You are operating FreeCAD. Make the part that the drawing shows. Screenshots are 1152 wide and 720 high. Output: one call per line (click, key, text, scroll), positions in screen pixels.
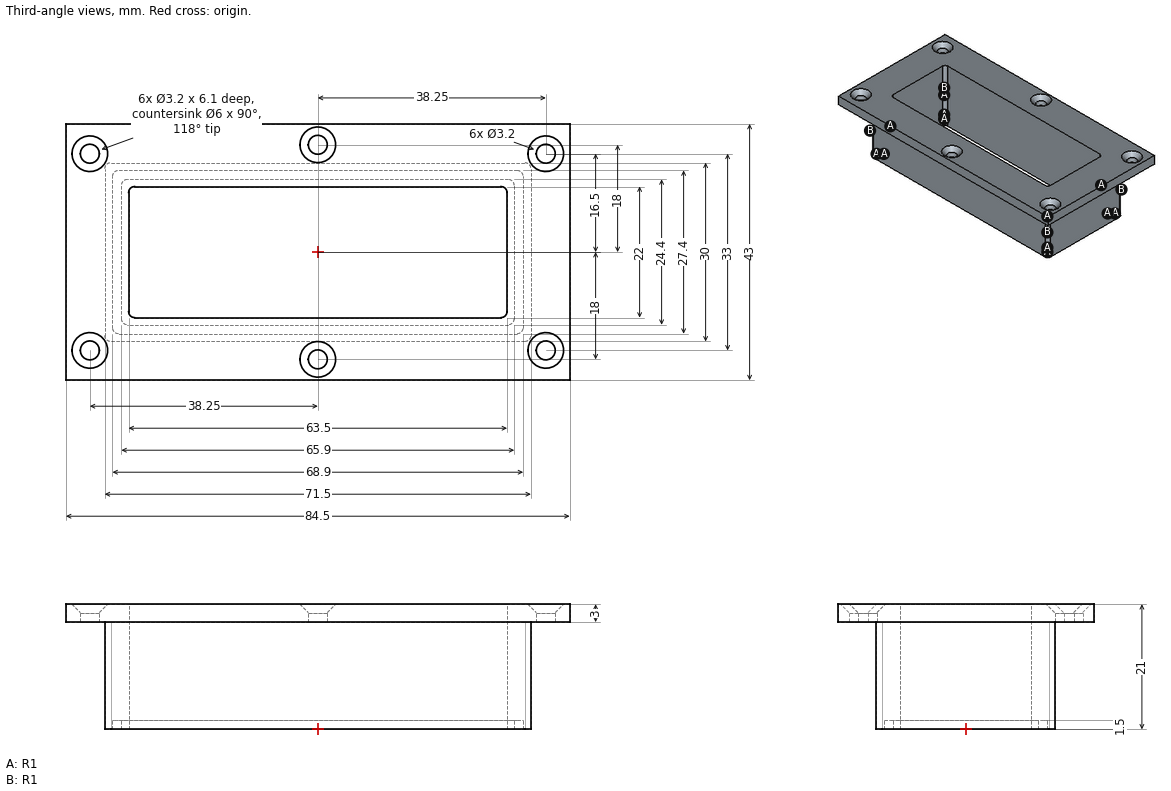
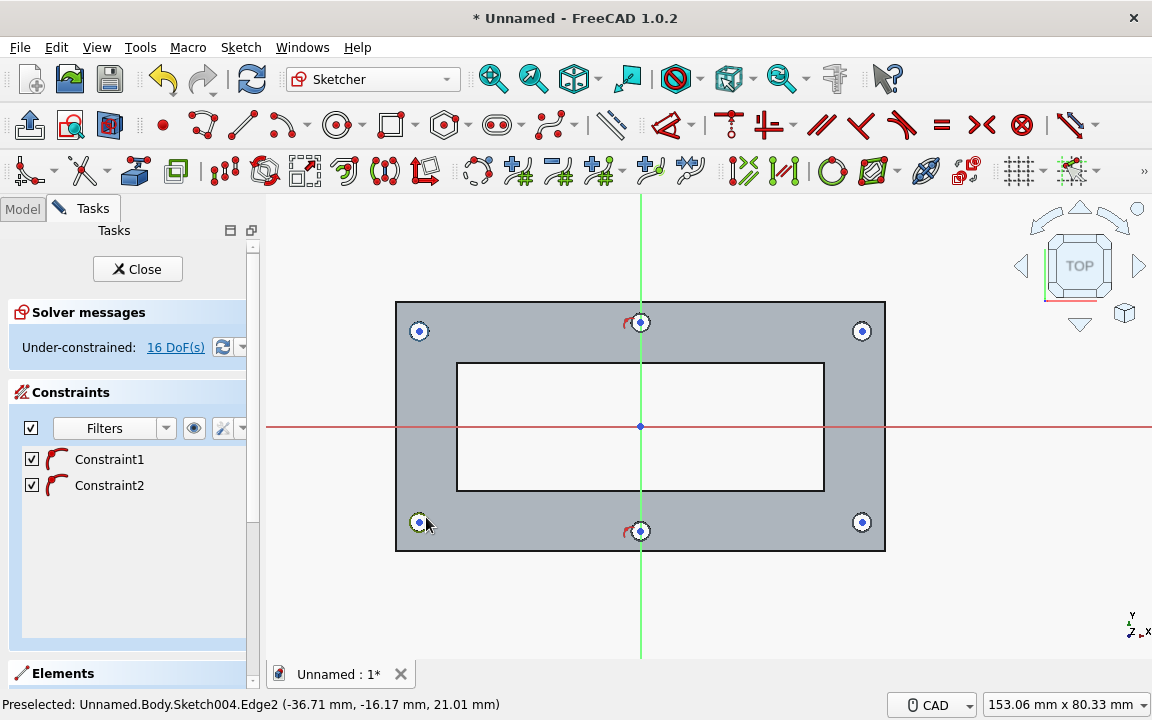
scroll(868, 325, up, 3)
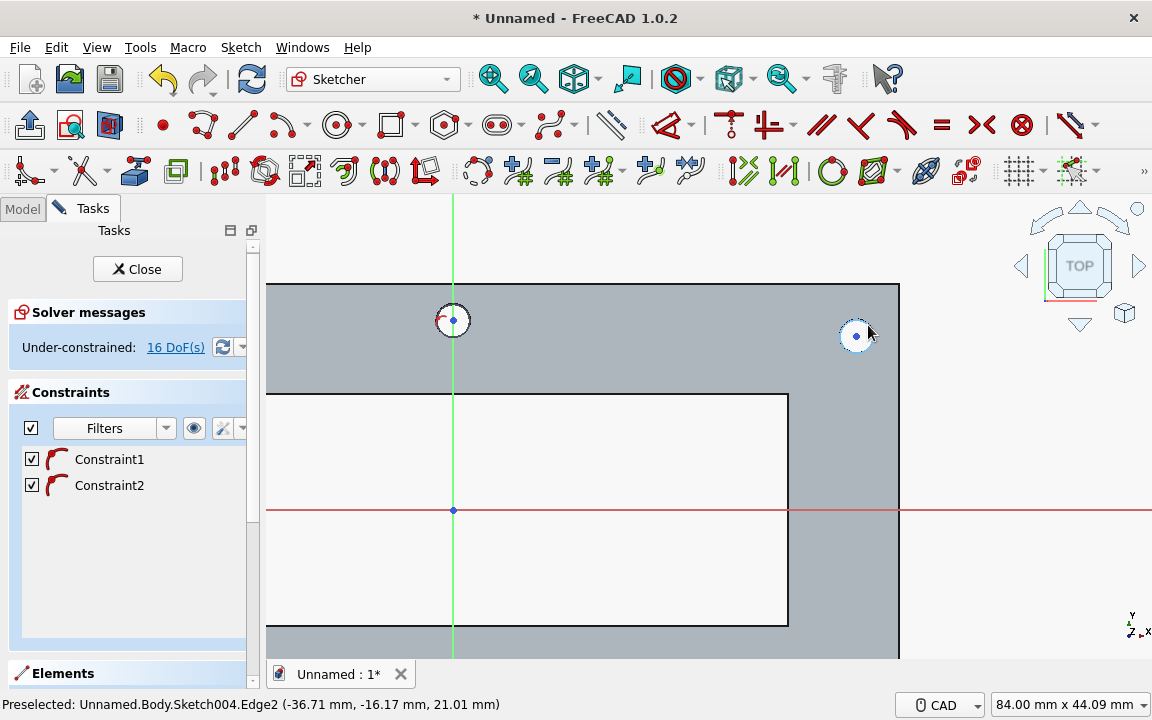
click(868, 325)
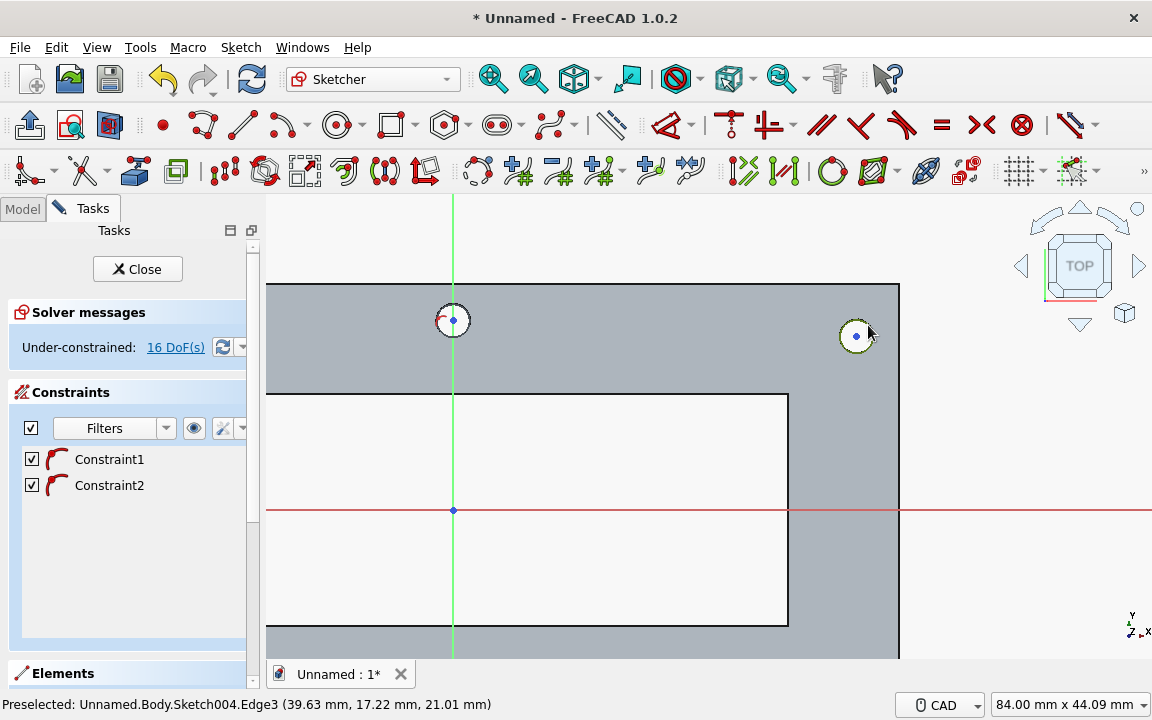
scroll(868, 325, down, 3)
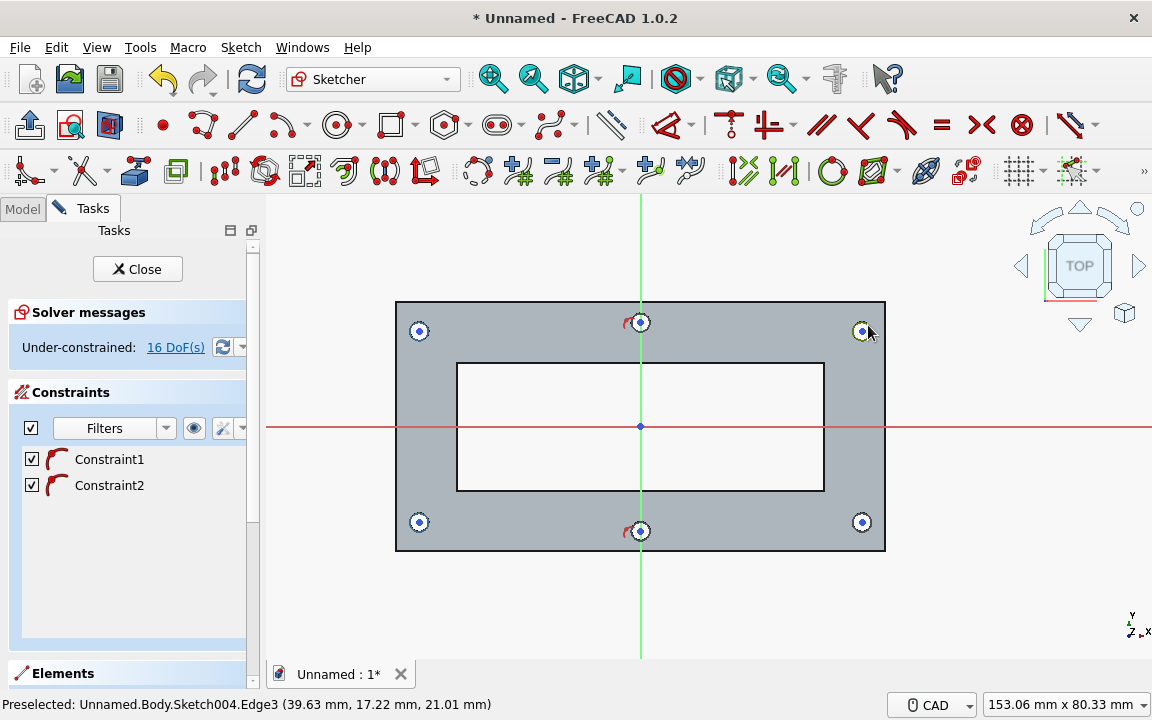
scroll(869, 516, up, 2)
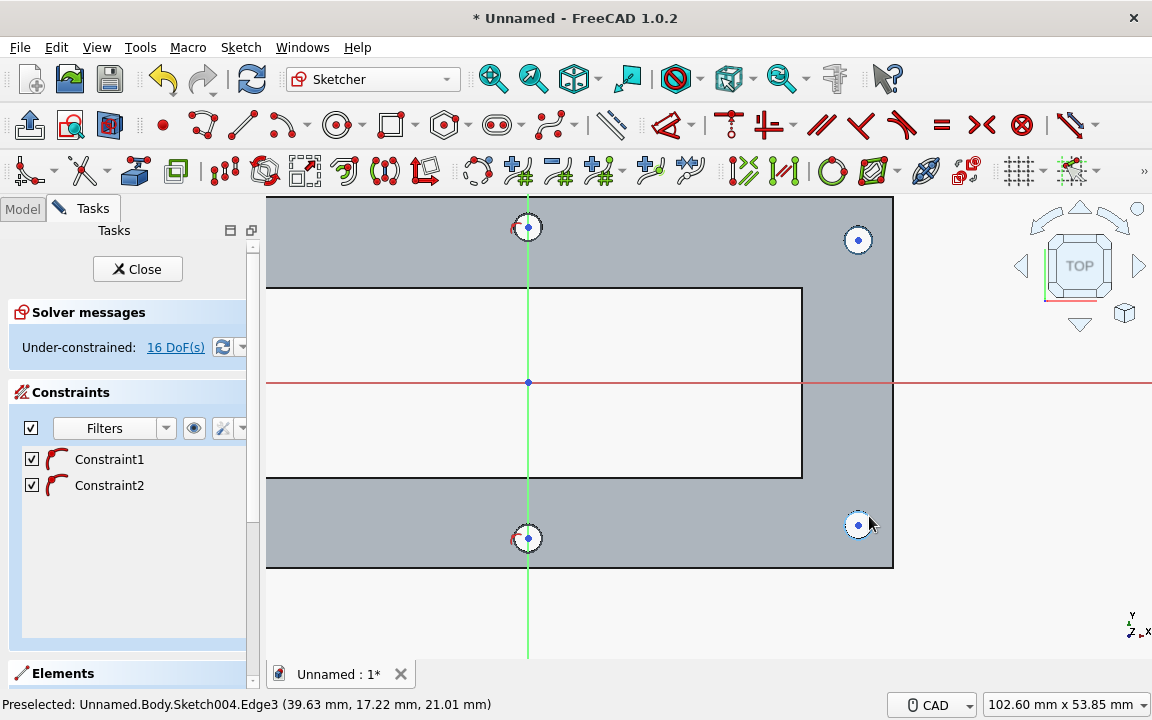
click(868, 516)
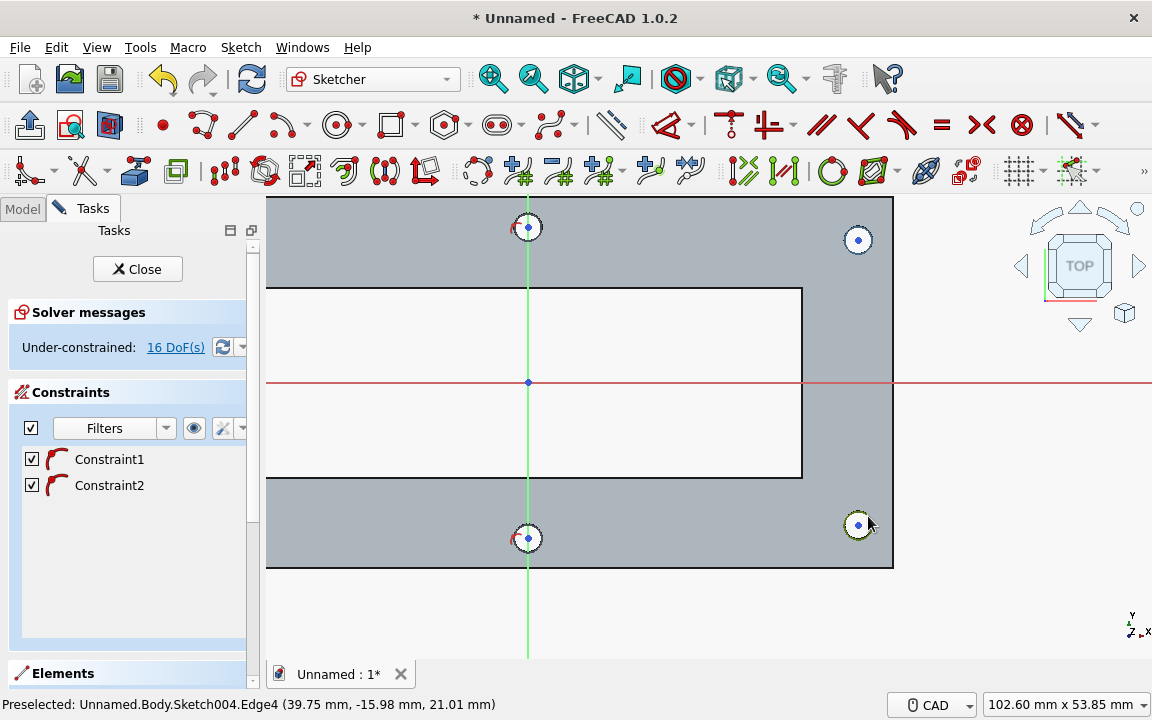
scroll(538, 529, up, 2)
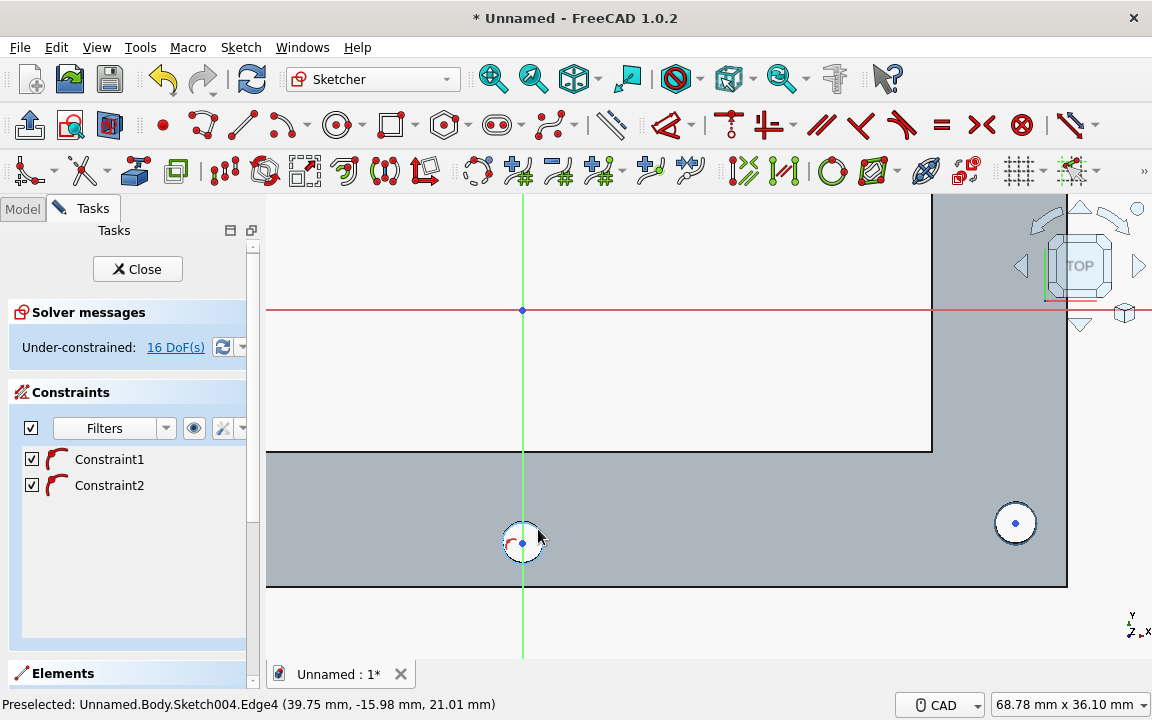
click(538, 529)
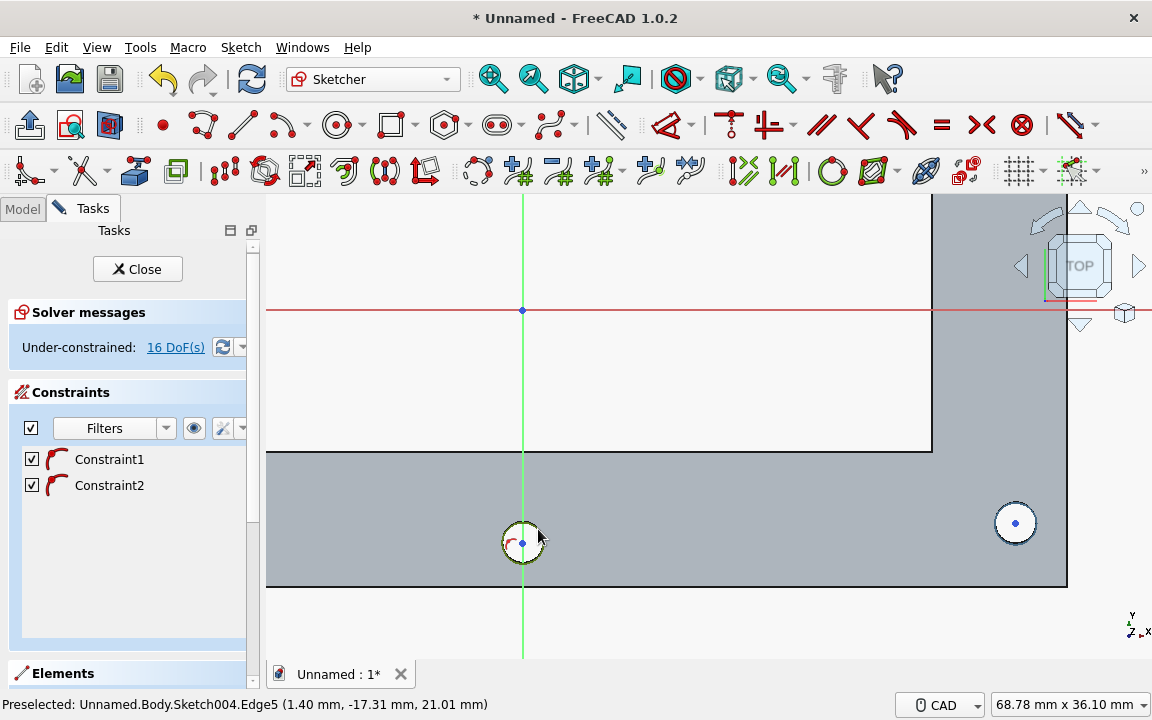
scroll(736, 521, down, 4)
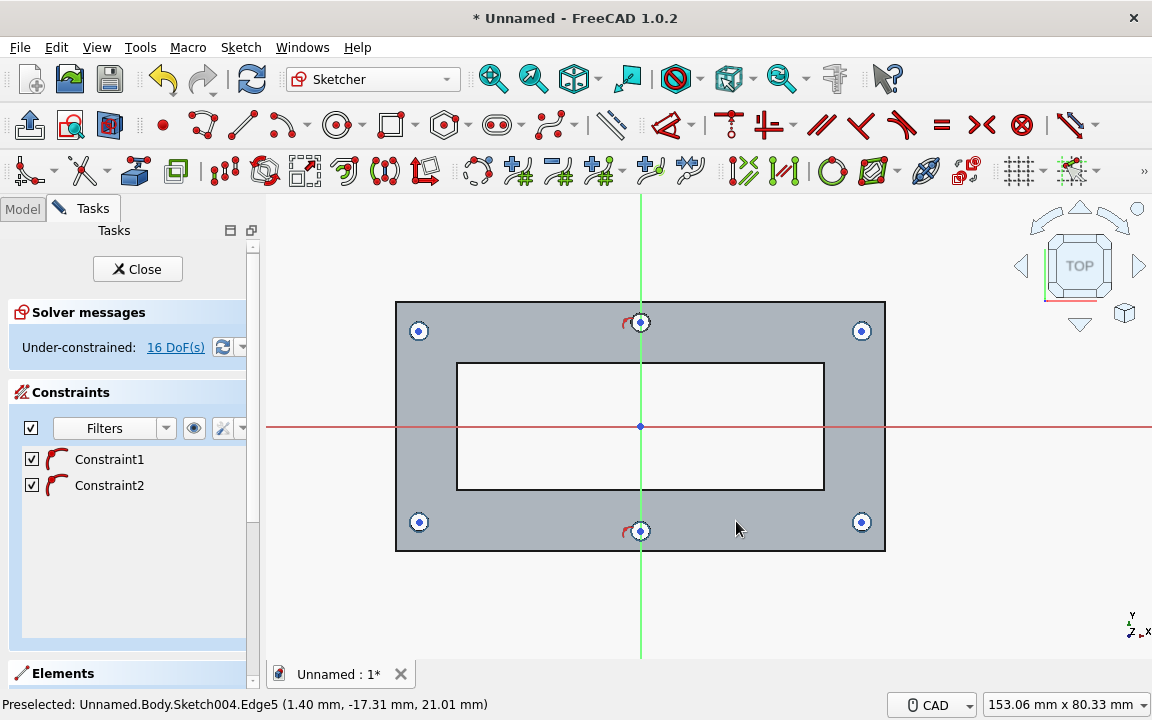
scroll(647, 316, up, 4)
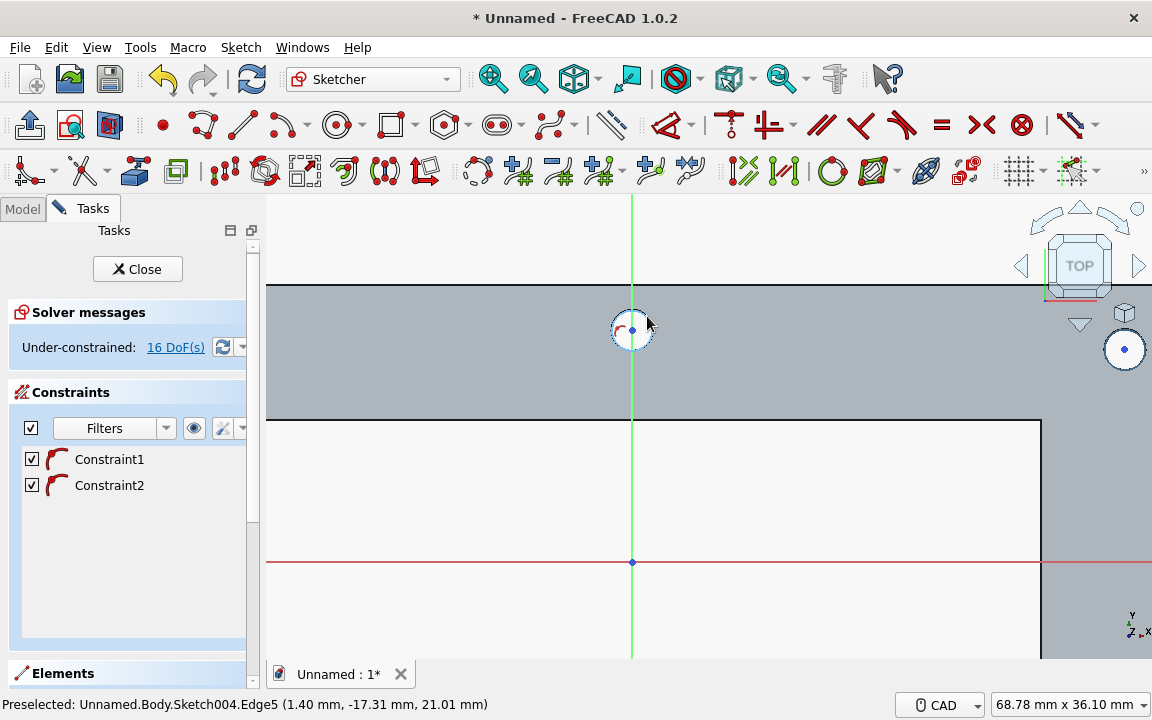
click(646, 316)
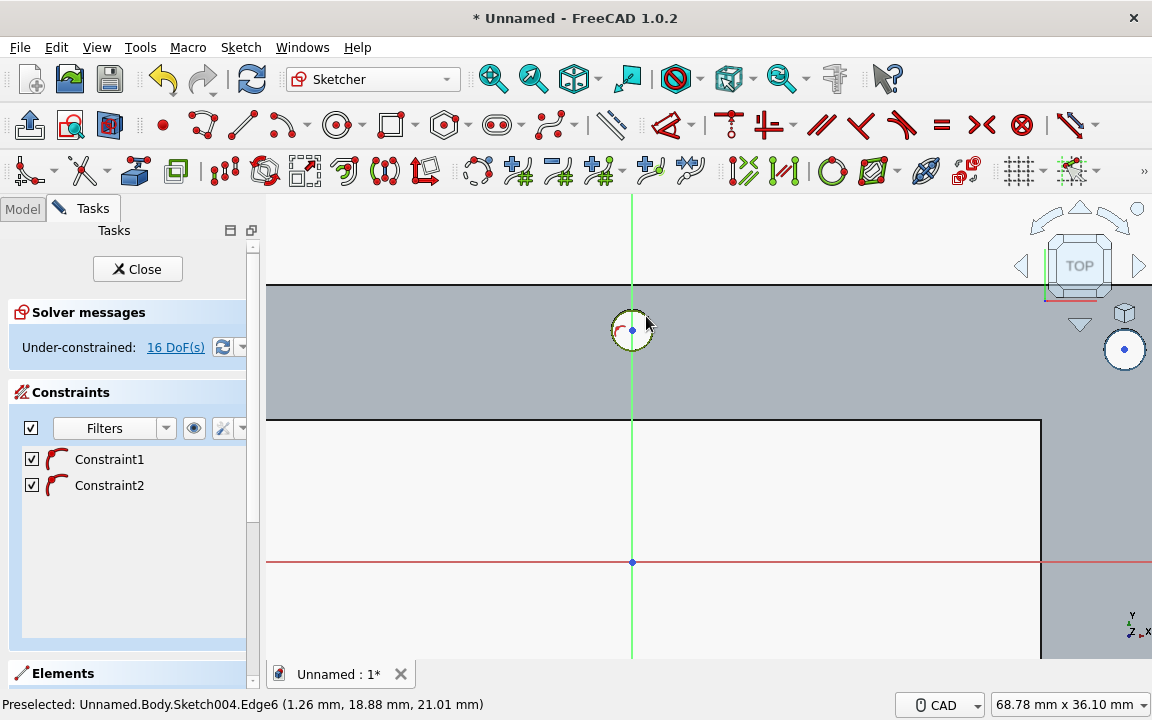
click(942, 126)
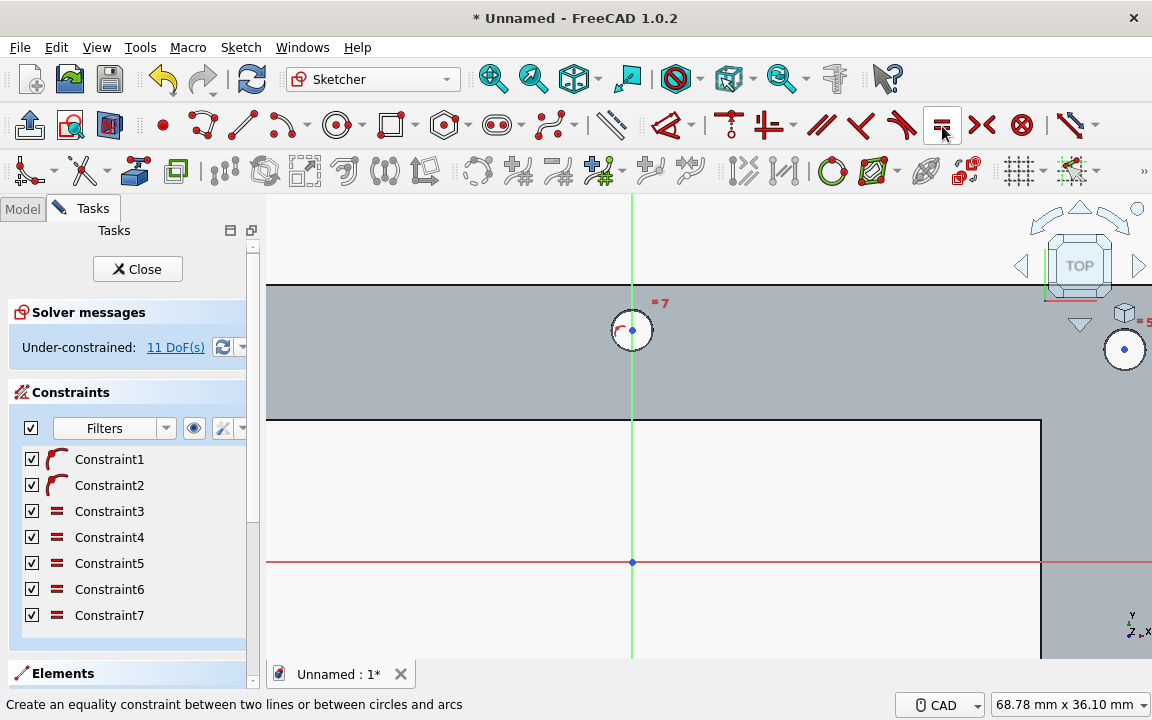
click(666, 126)